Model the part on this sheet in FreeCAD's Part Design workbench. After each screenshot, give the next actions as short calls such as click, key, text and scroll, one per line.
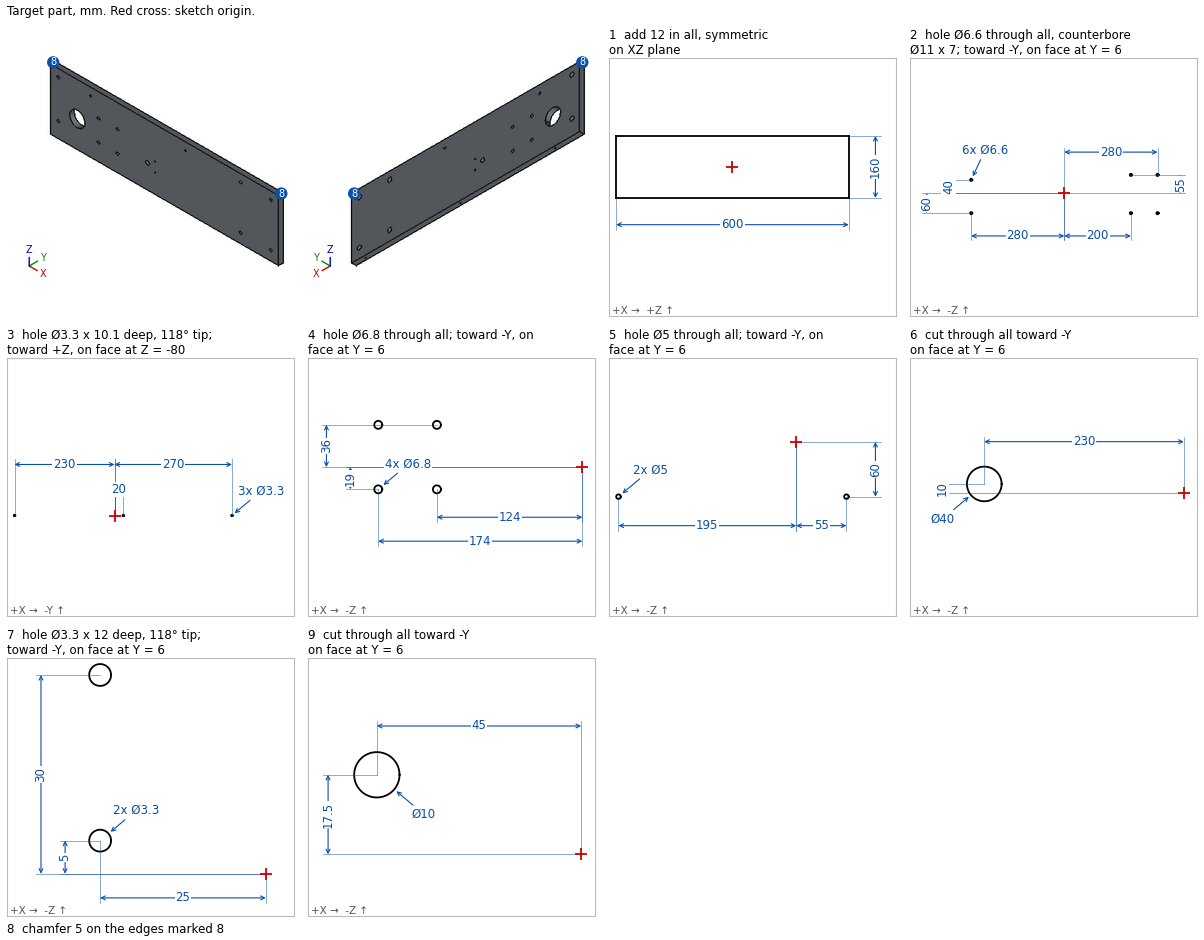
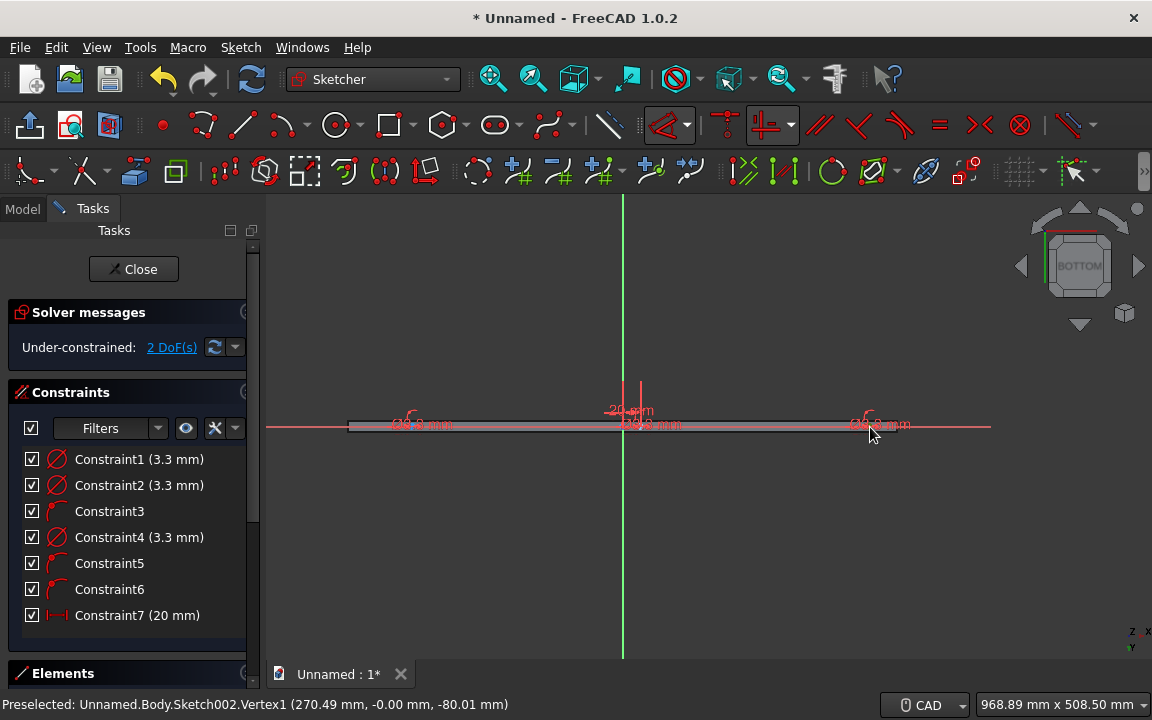
click(690, 126)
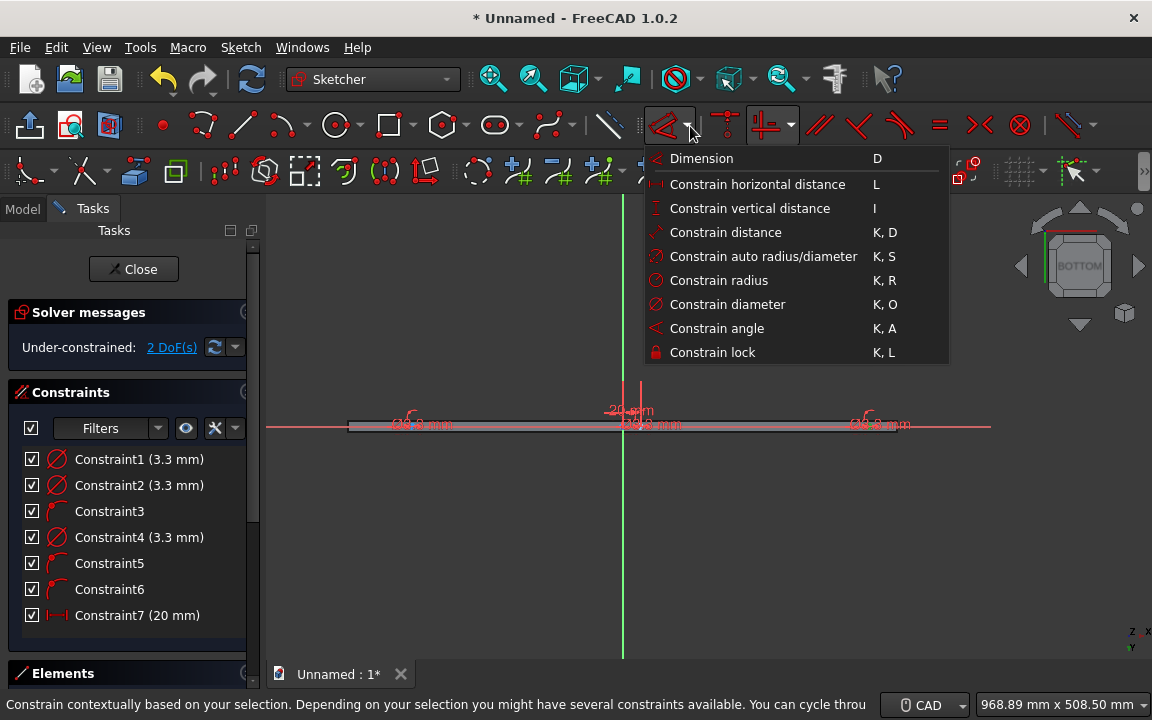
click(797, 184)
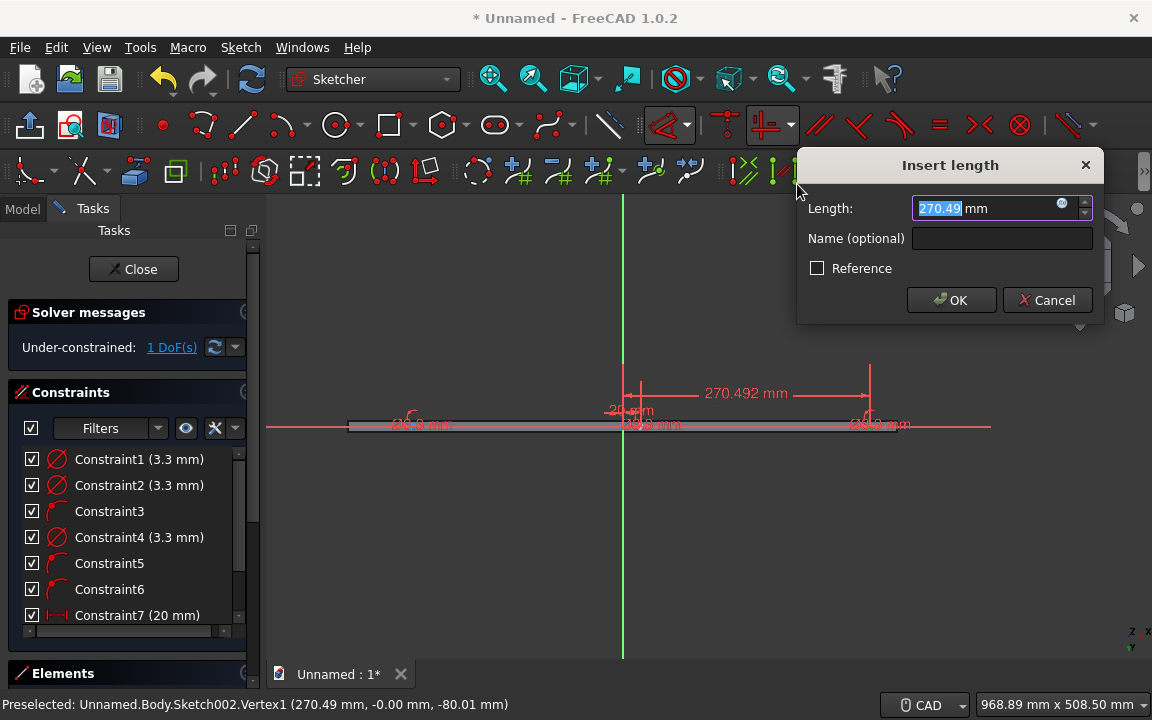
text(270)
key(Return)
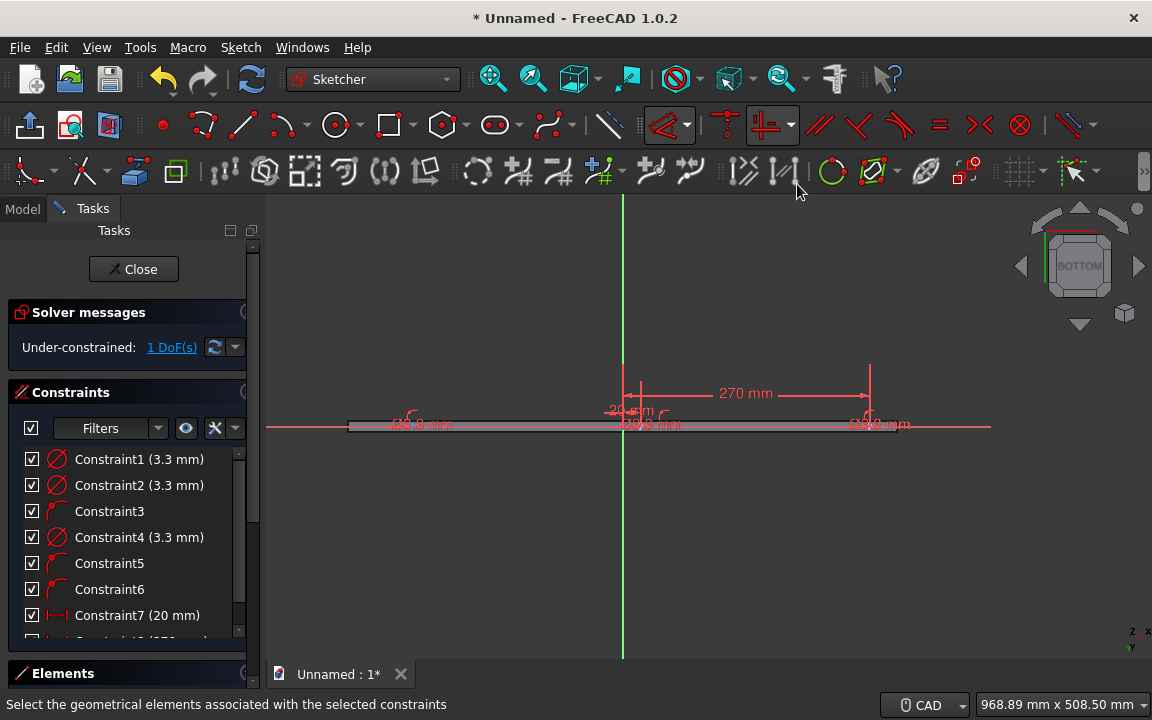
click(412, 427)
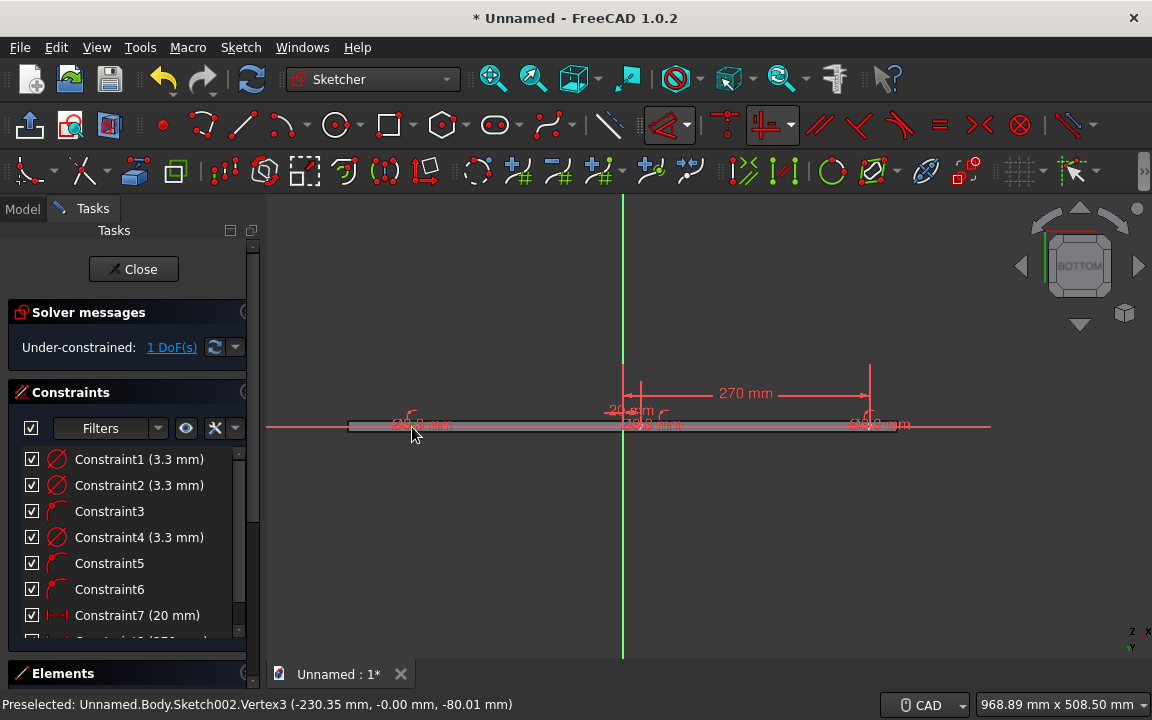
click(690, 126)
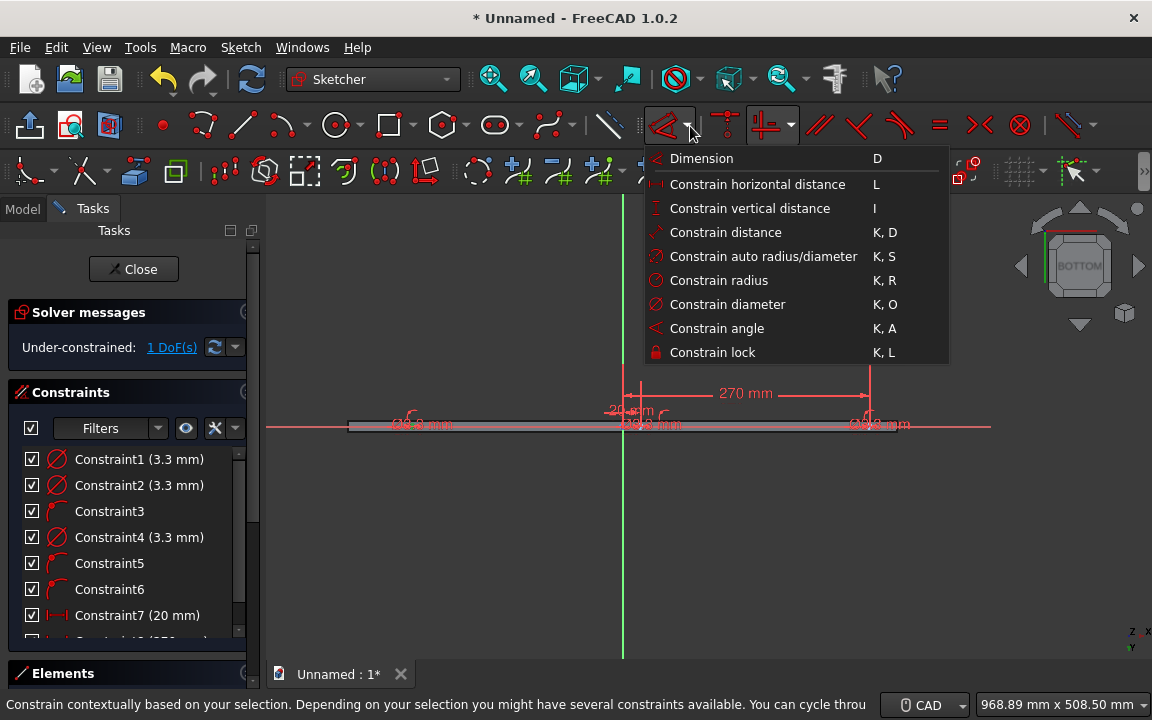
click(797, 184)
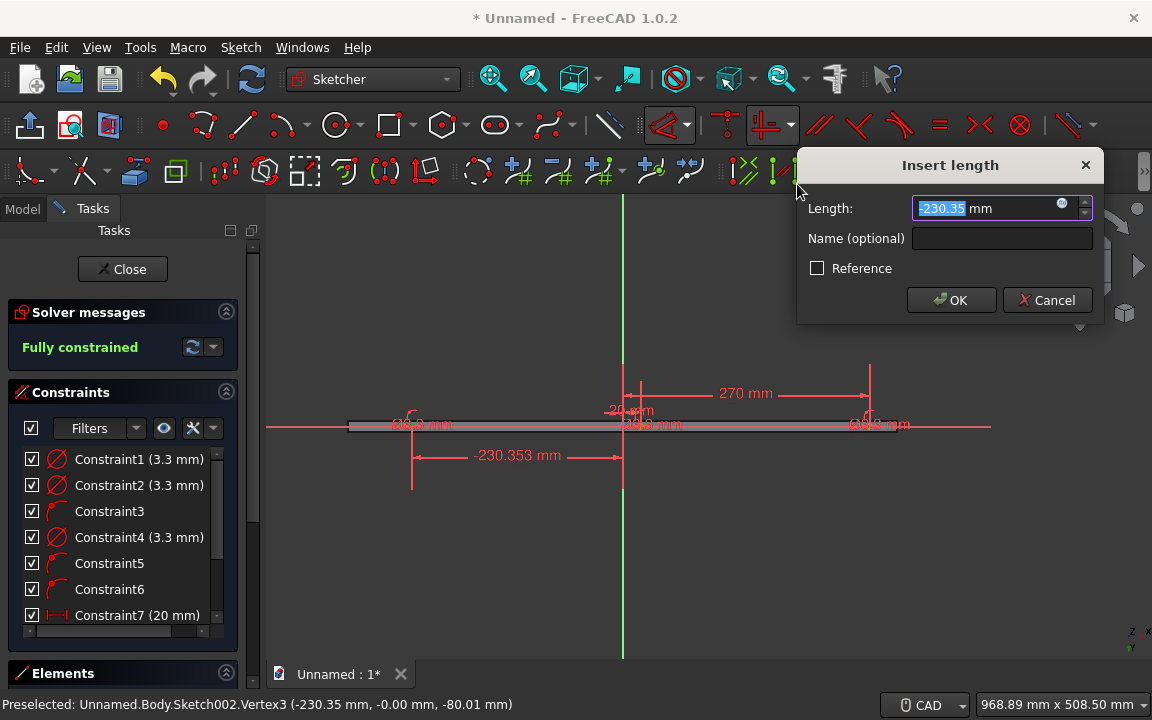
text(-230)
key(Return)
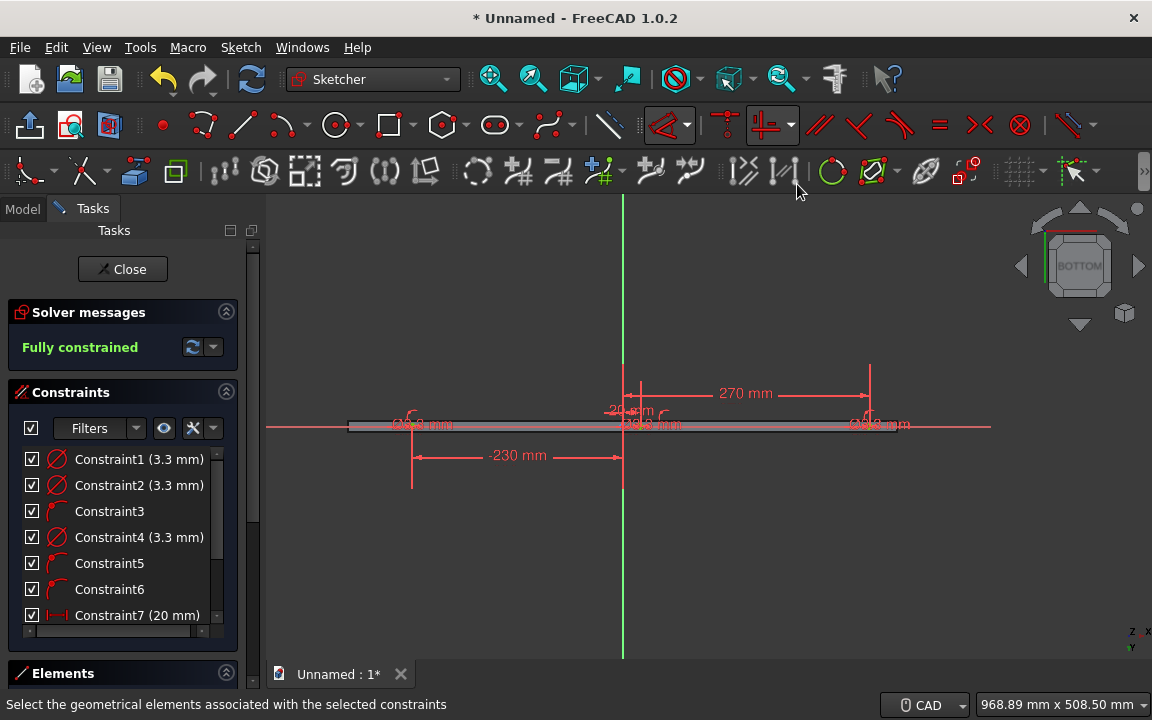
click(123, 269)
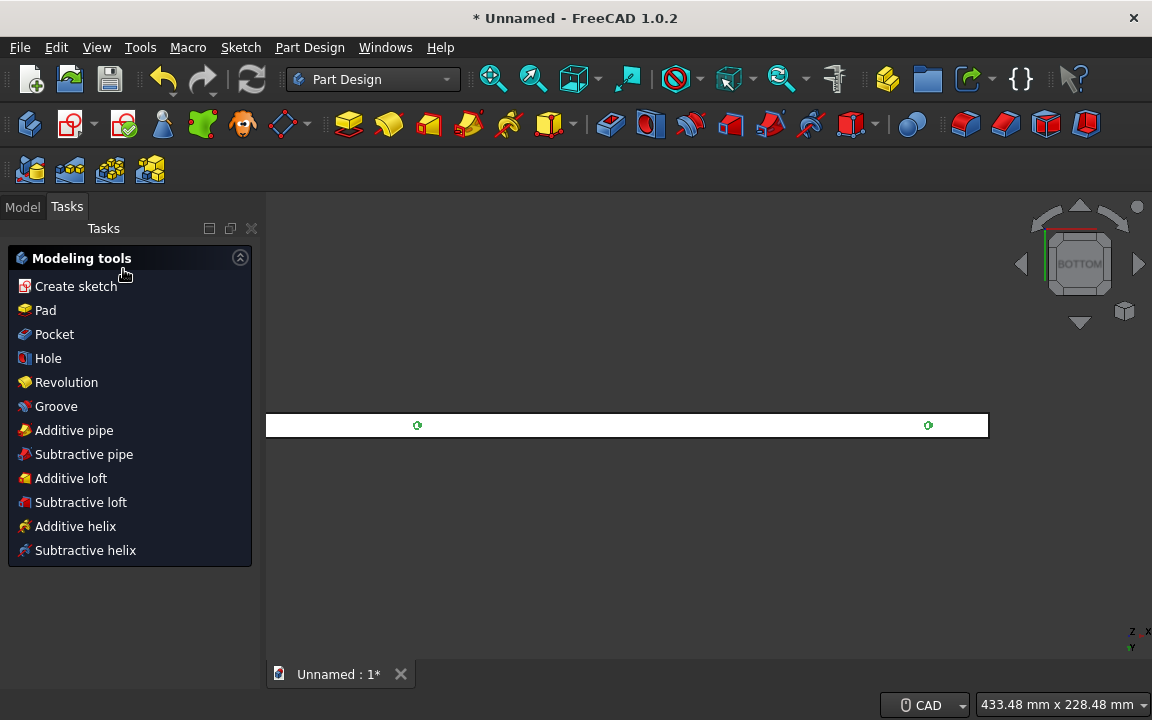
click(652, 124)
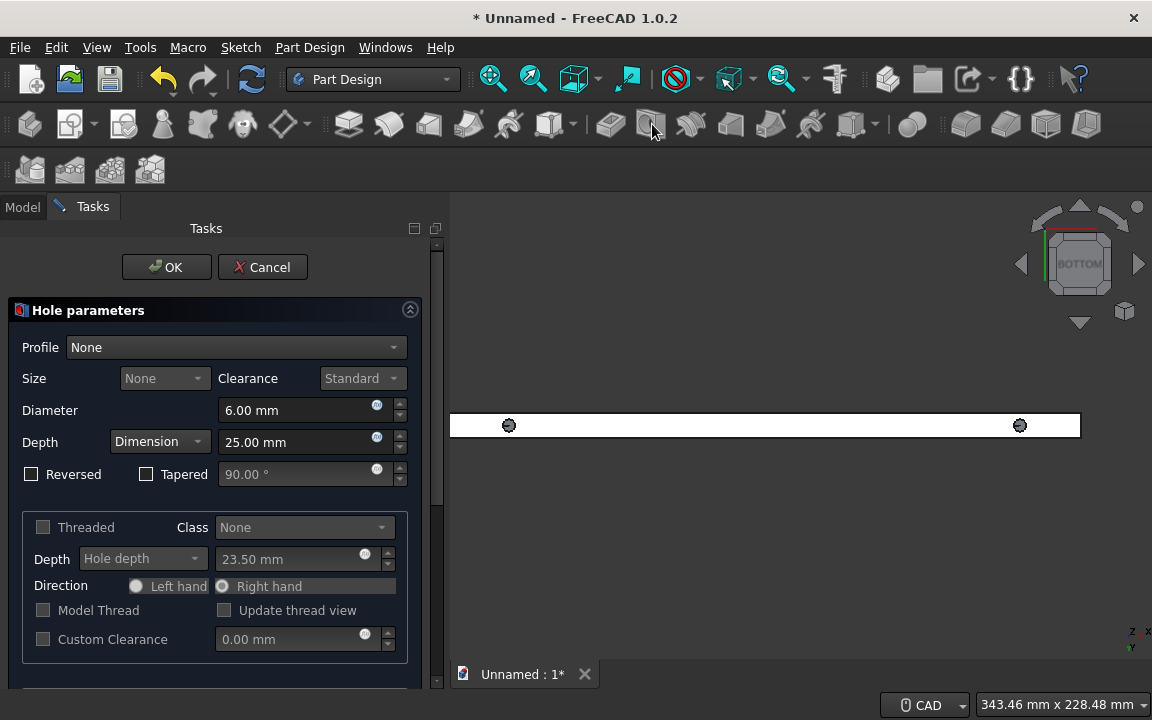
triple_click(305, 410)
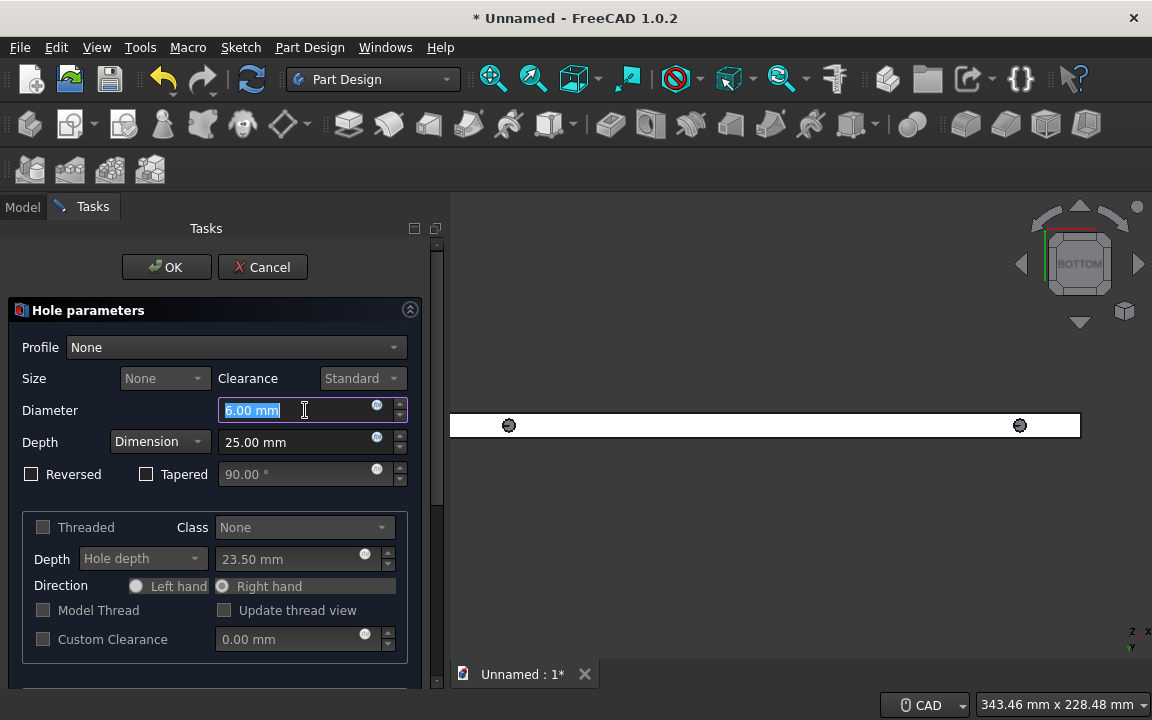
text(3.3)
key(Tab)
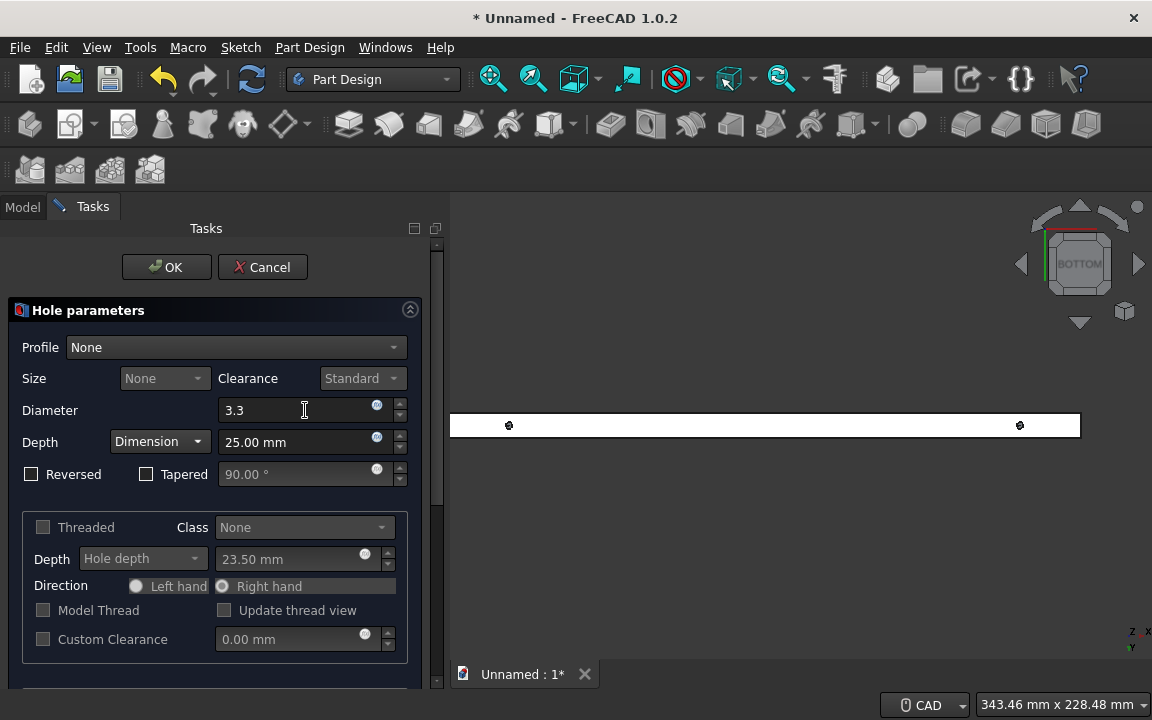
triple_click(305, 442)